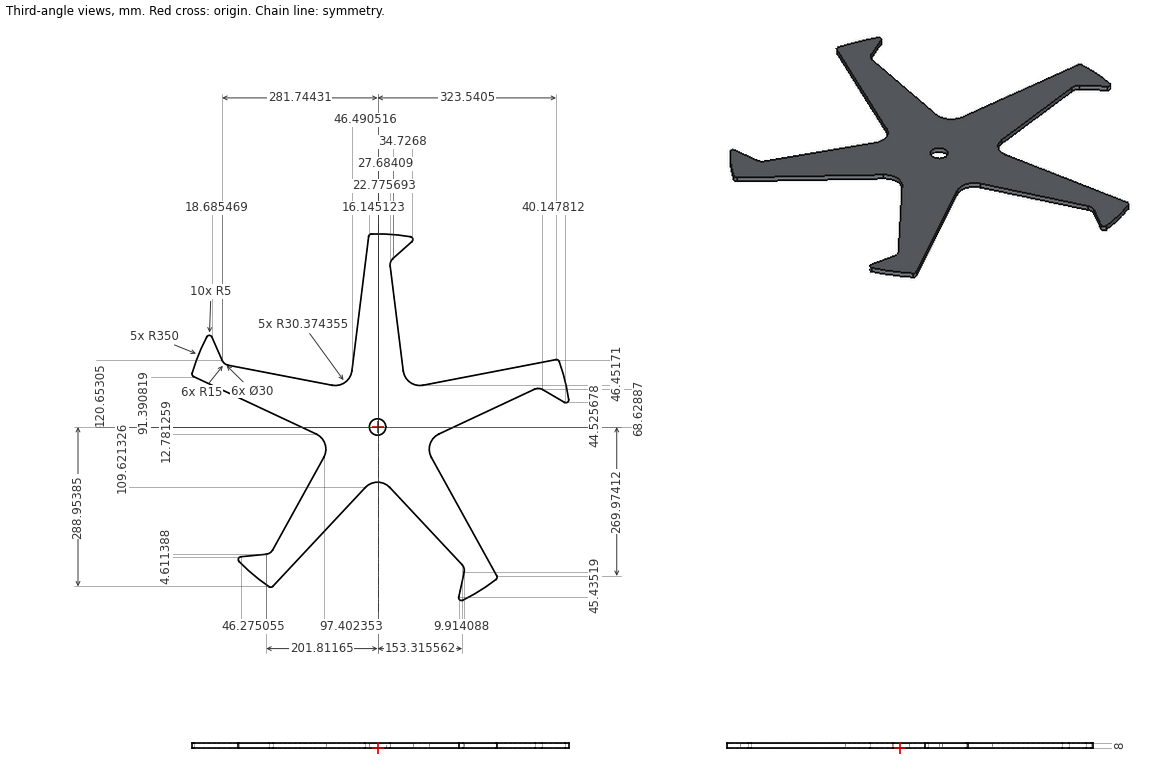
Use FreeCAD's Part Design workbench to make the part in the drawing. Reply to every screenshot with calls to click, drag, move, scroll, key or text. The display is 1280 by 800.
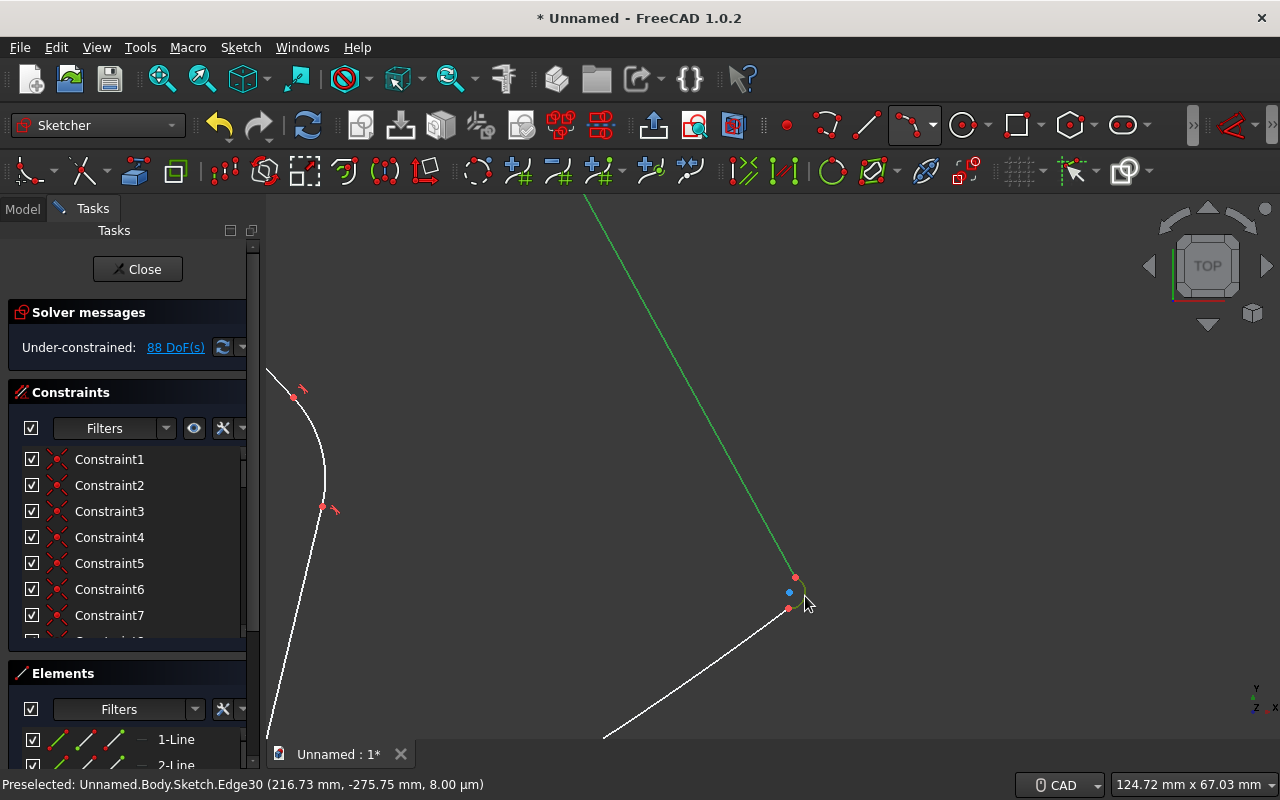
key(t)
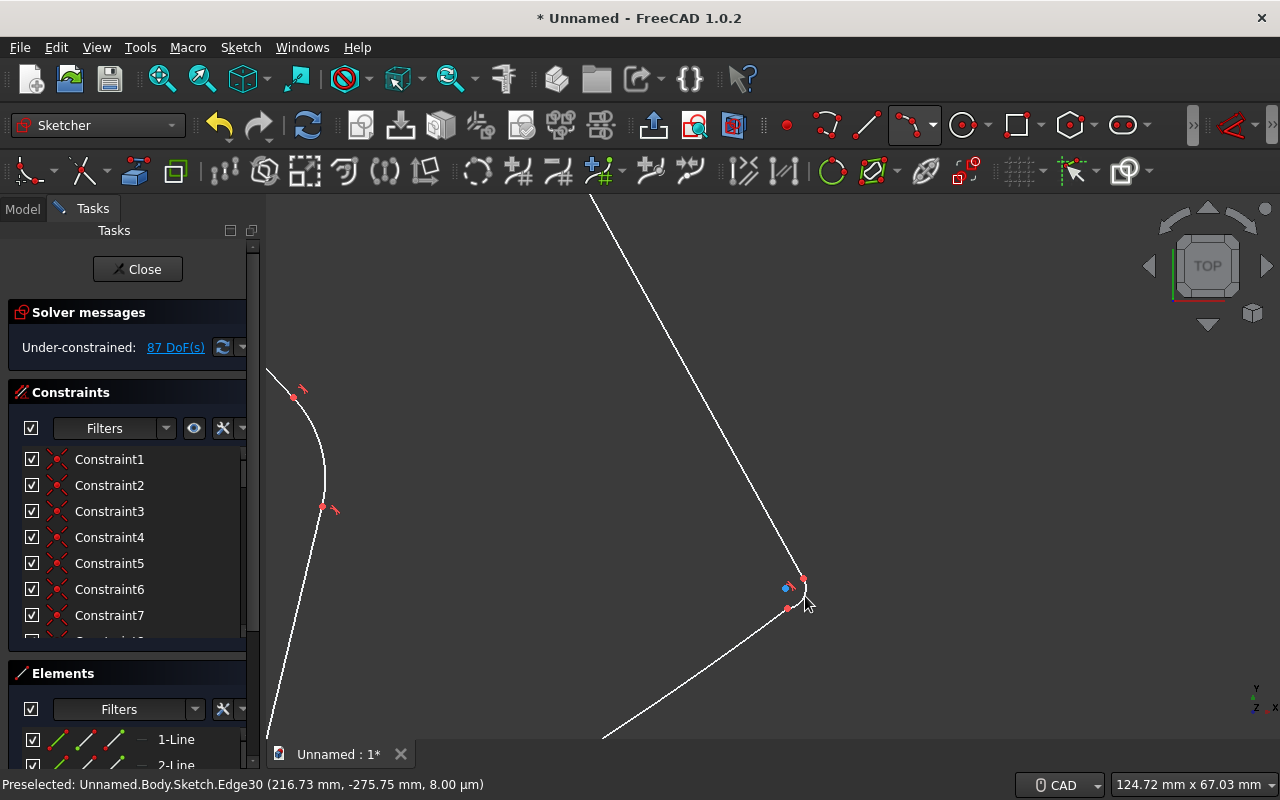
scroll(810, 612, down, 14)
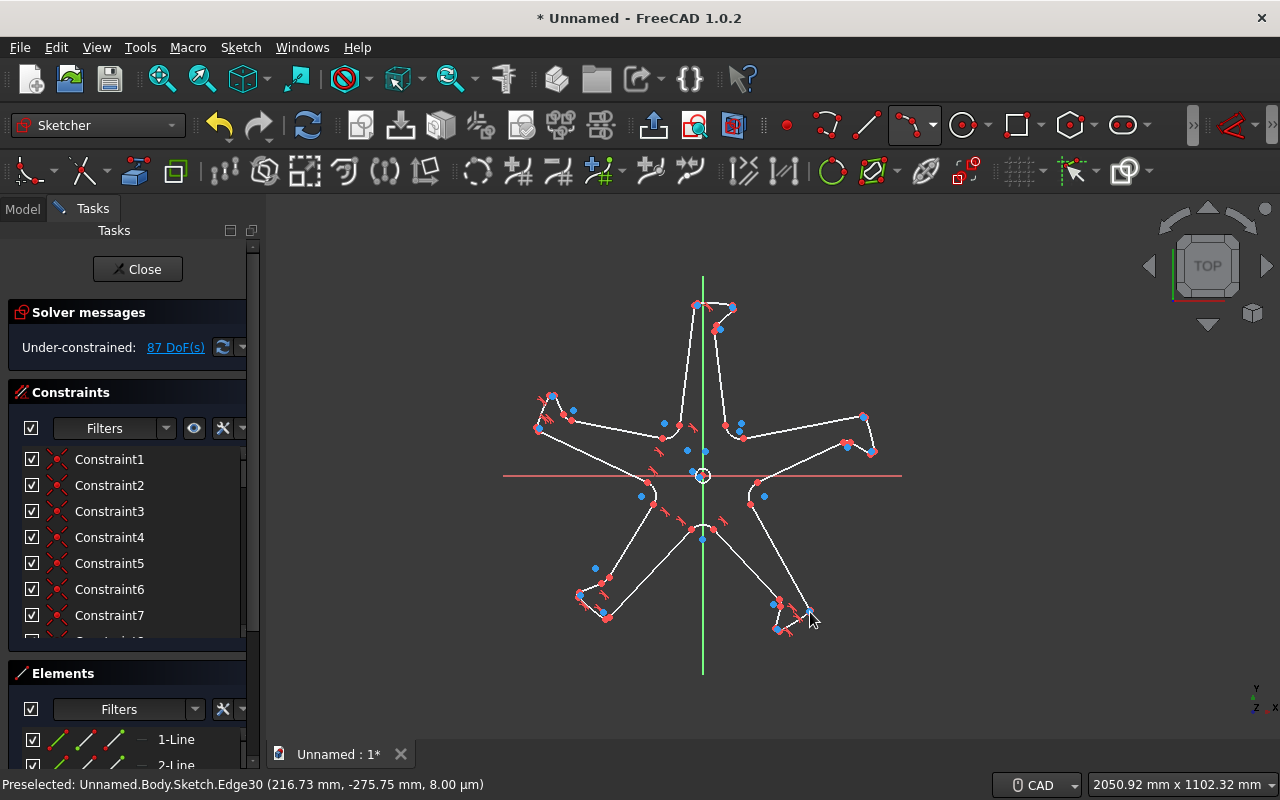
click(798, 589)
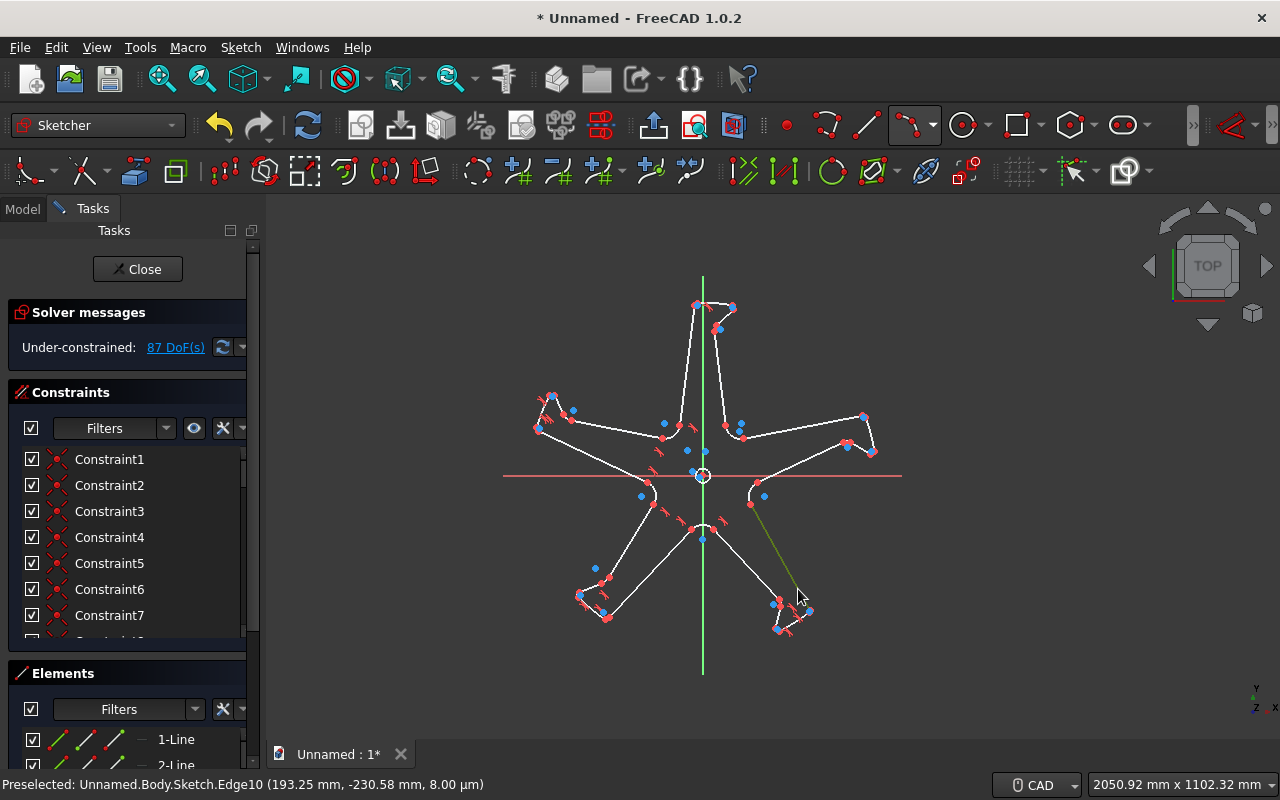
click(750, 492)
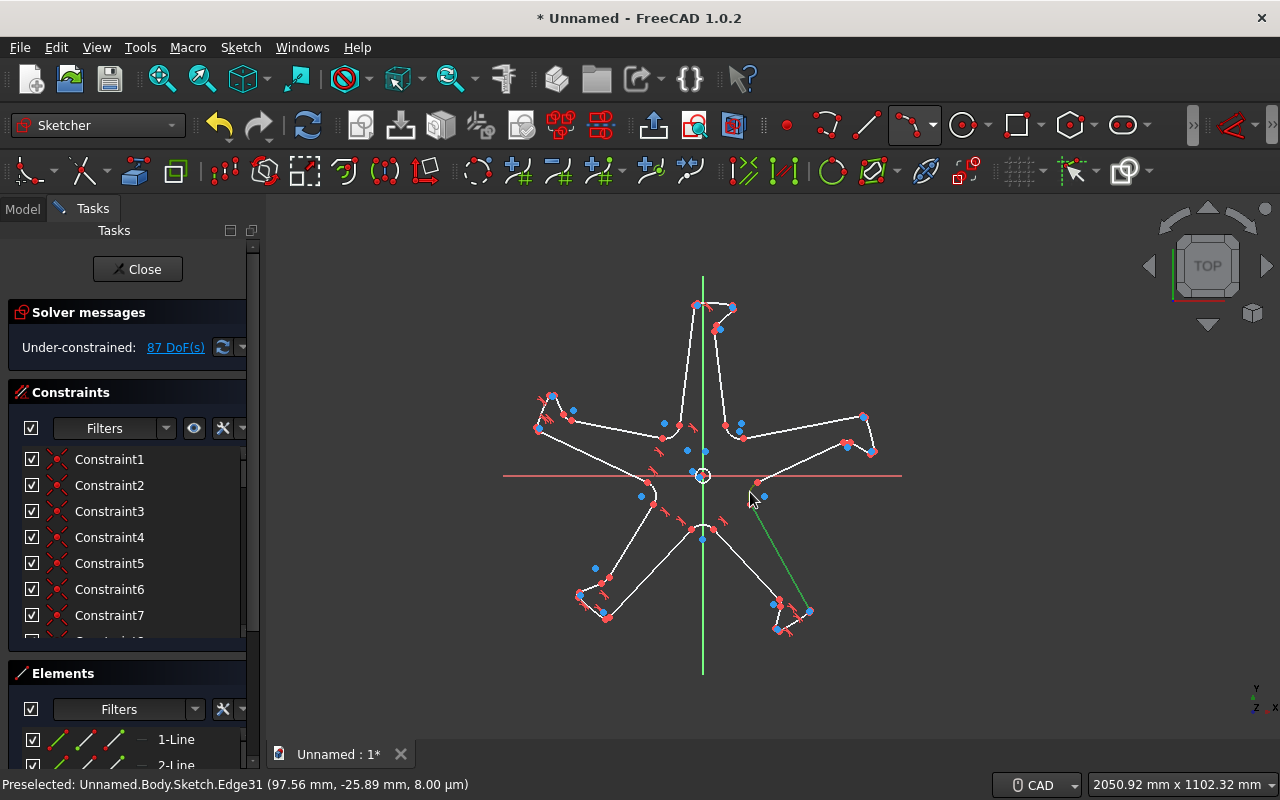
key(t)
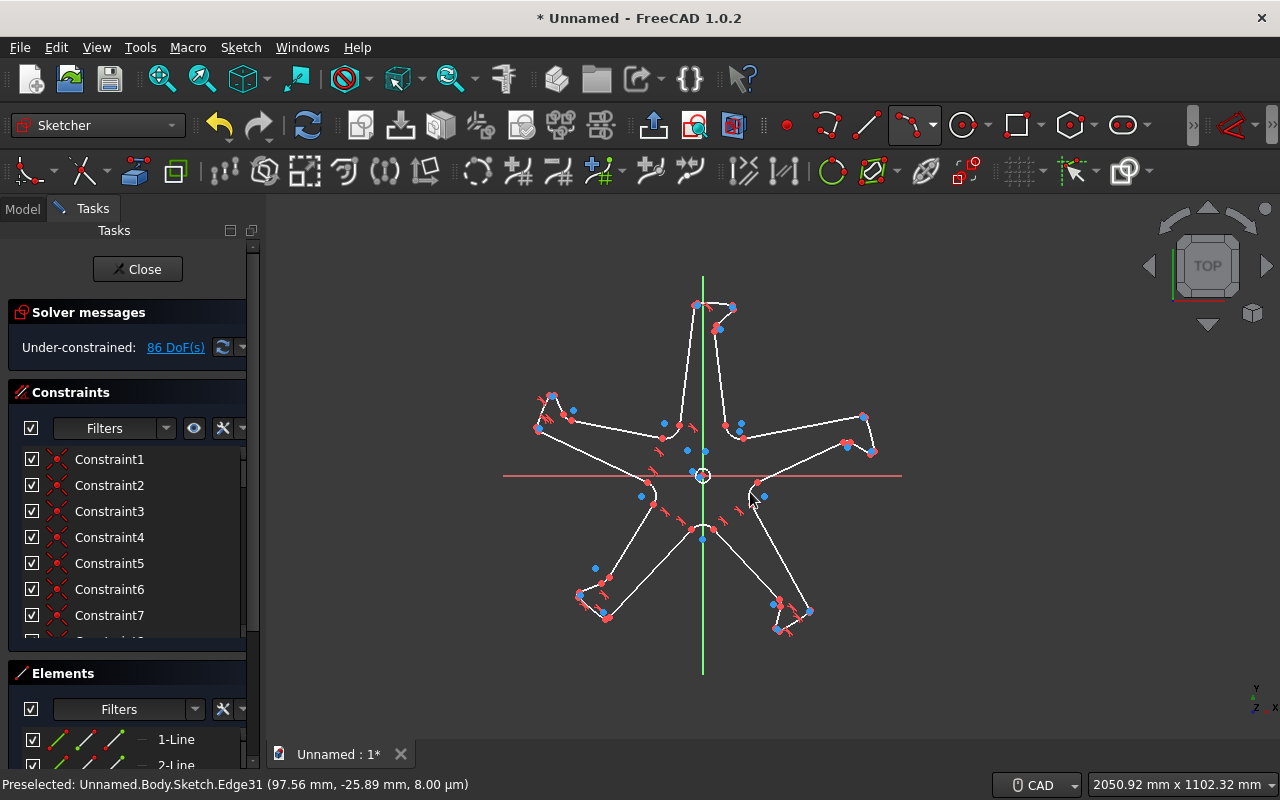
click(818, 454)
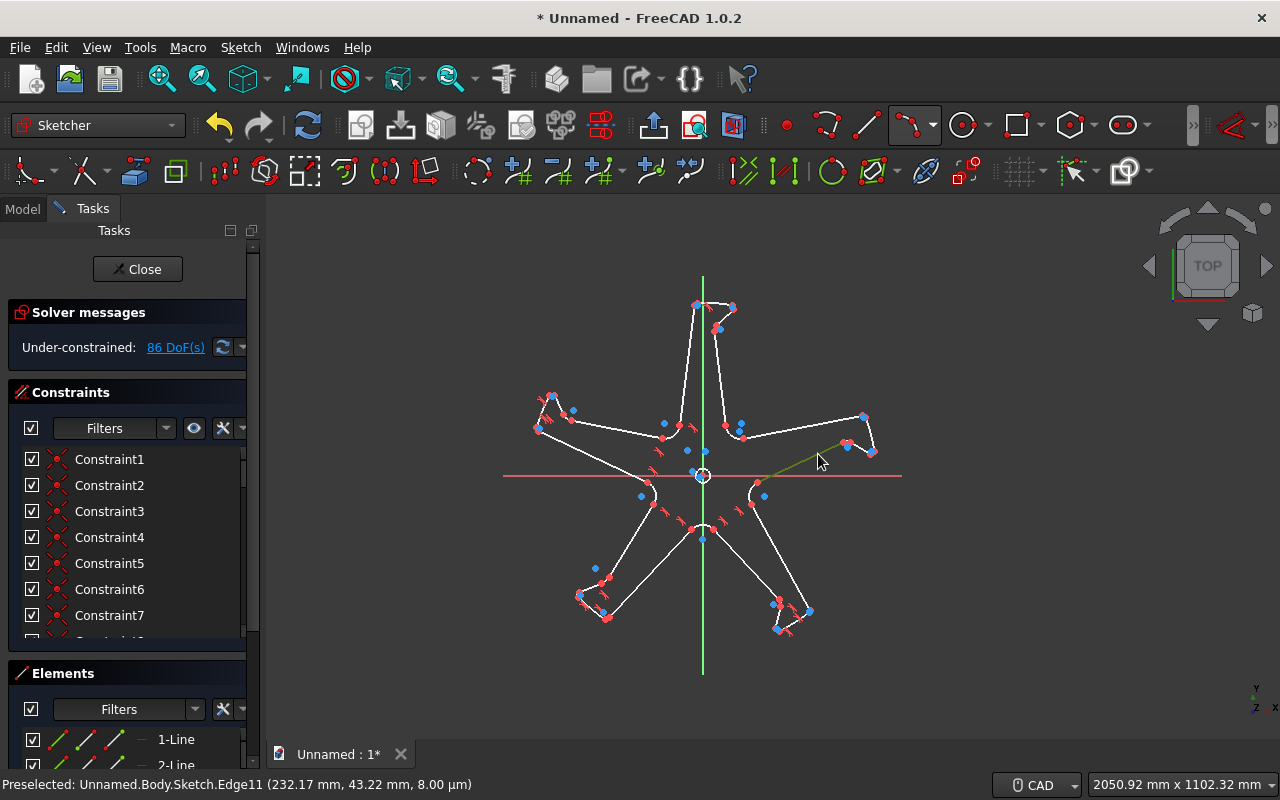
click(750, 492)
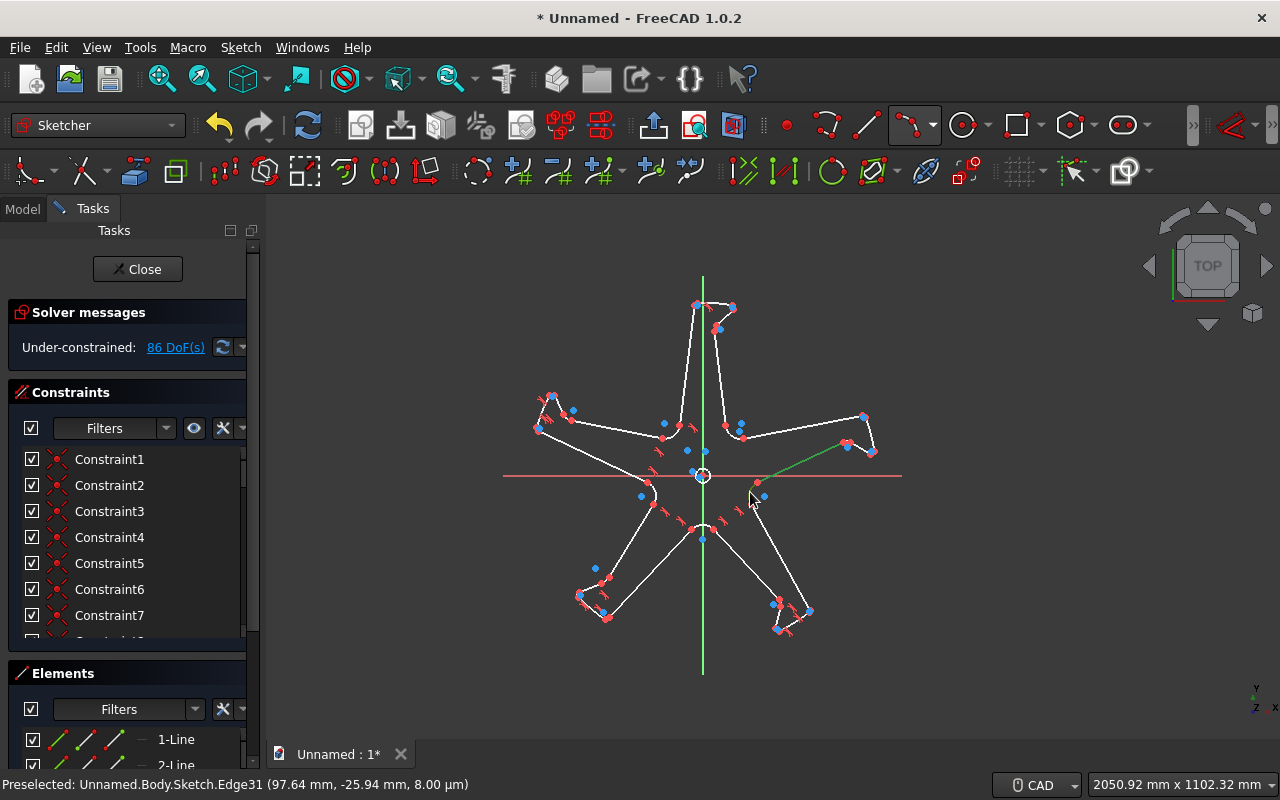
key(t)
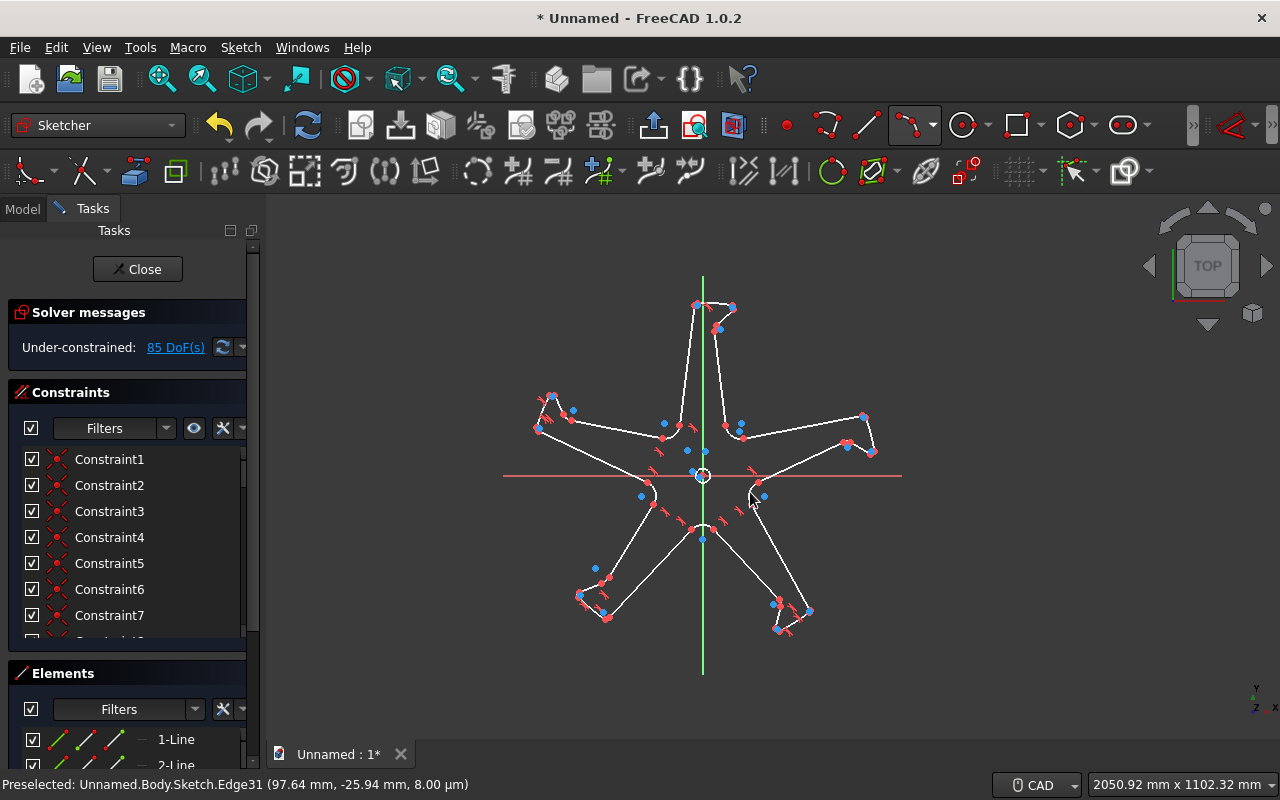
click(818, 454)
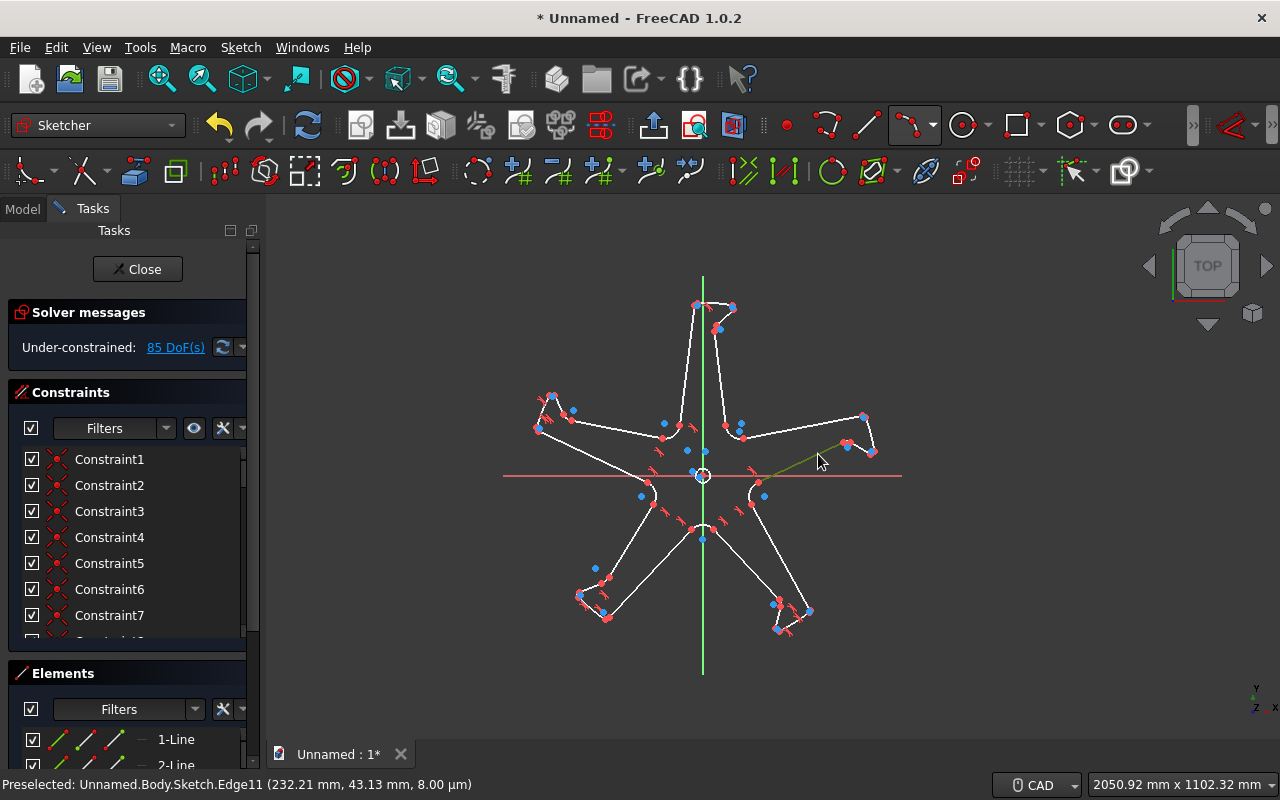
scroll(847, 441, up, 7)